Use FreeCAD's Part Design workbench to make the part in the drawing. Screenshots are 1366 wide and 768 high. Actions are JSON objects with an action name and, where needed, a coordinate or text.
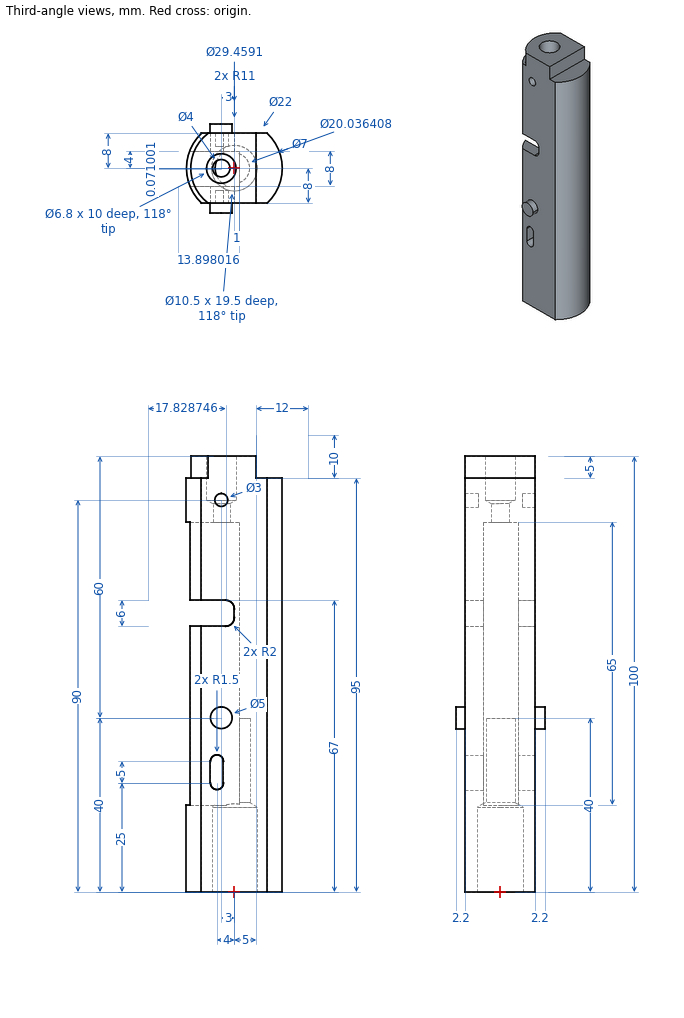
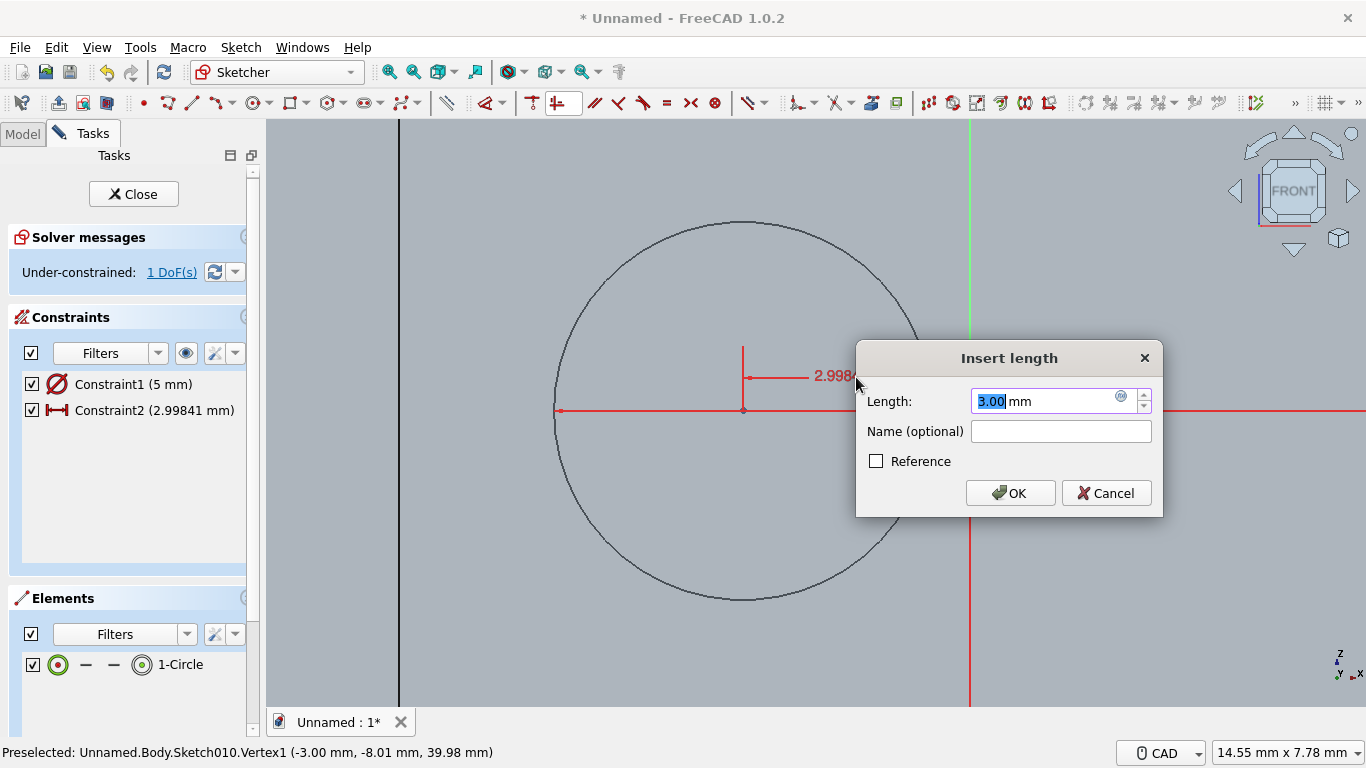
{"action": "type", "text": "3"}
{"action": "key", "text": "Return"}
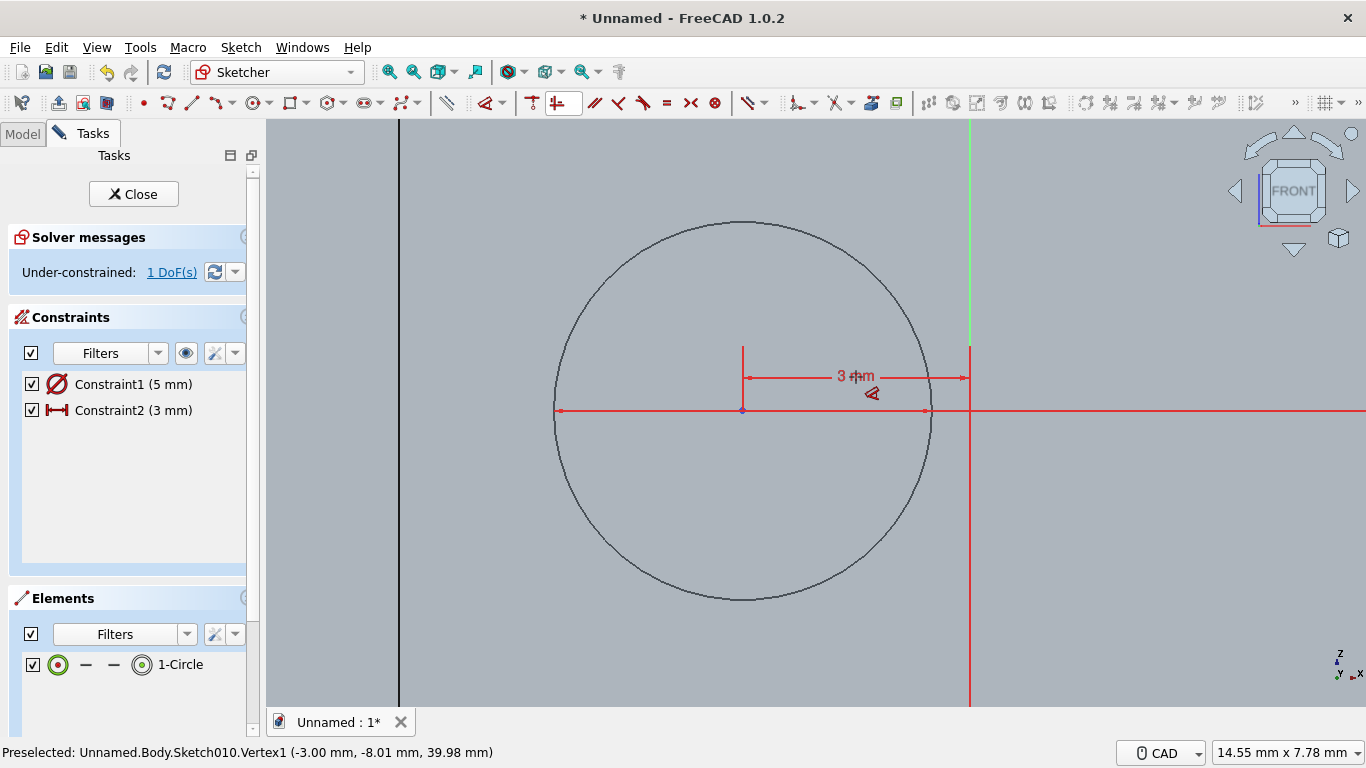
{"action": "left_click", "coordinate": [743, 411]}
{"action": "left_click", "coordinate": [1004, 545]}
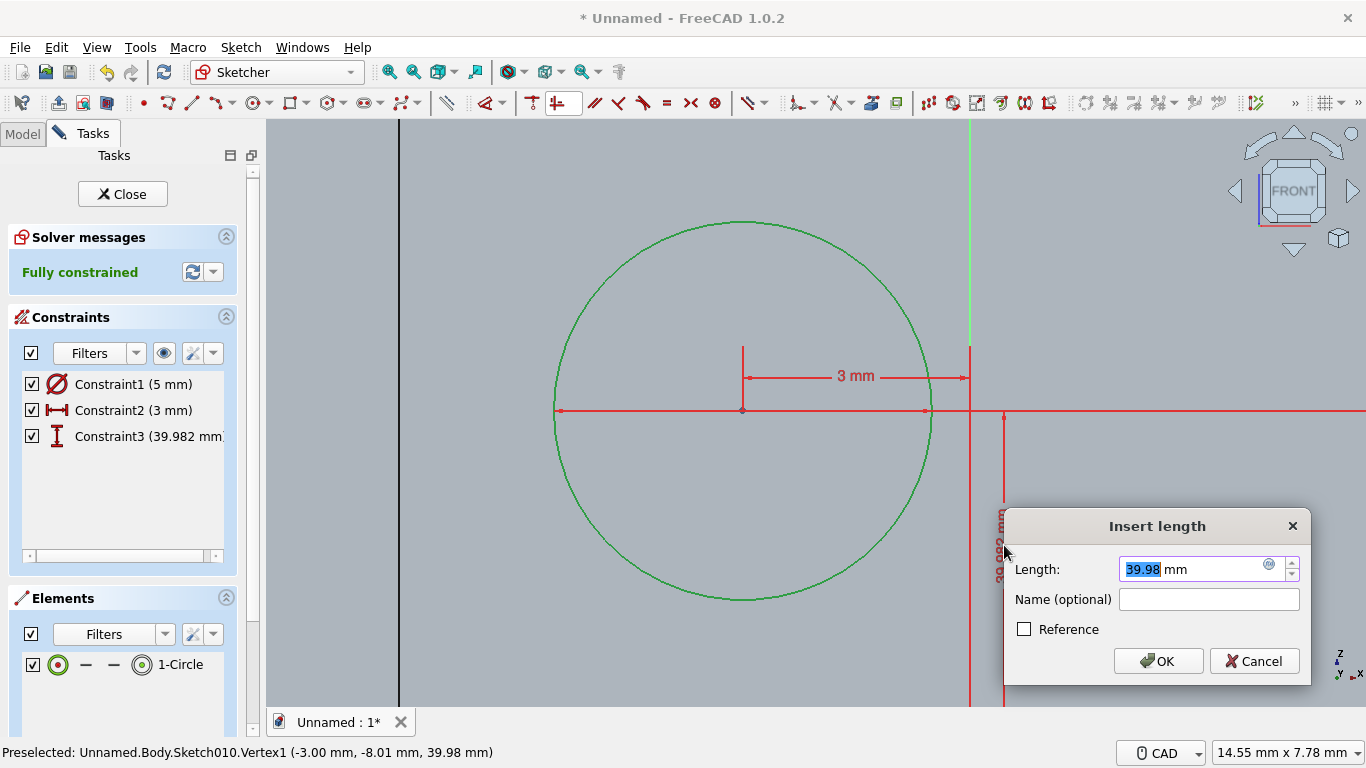
{"action": "type", "text": "40"}
{"action": "key", "text": "Return"}
{"action": "key", "text": "Escape"}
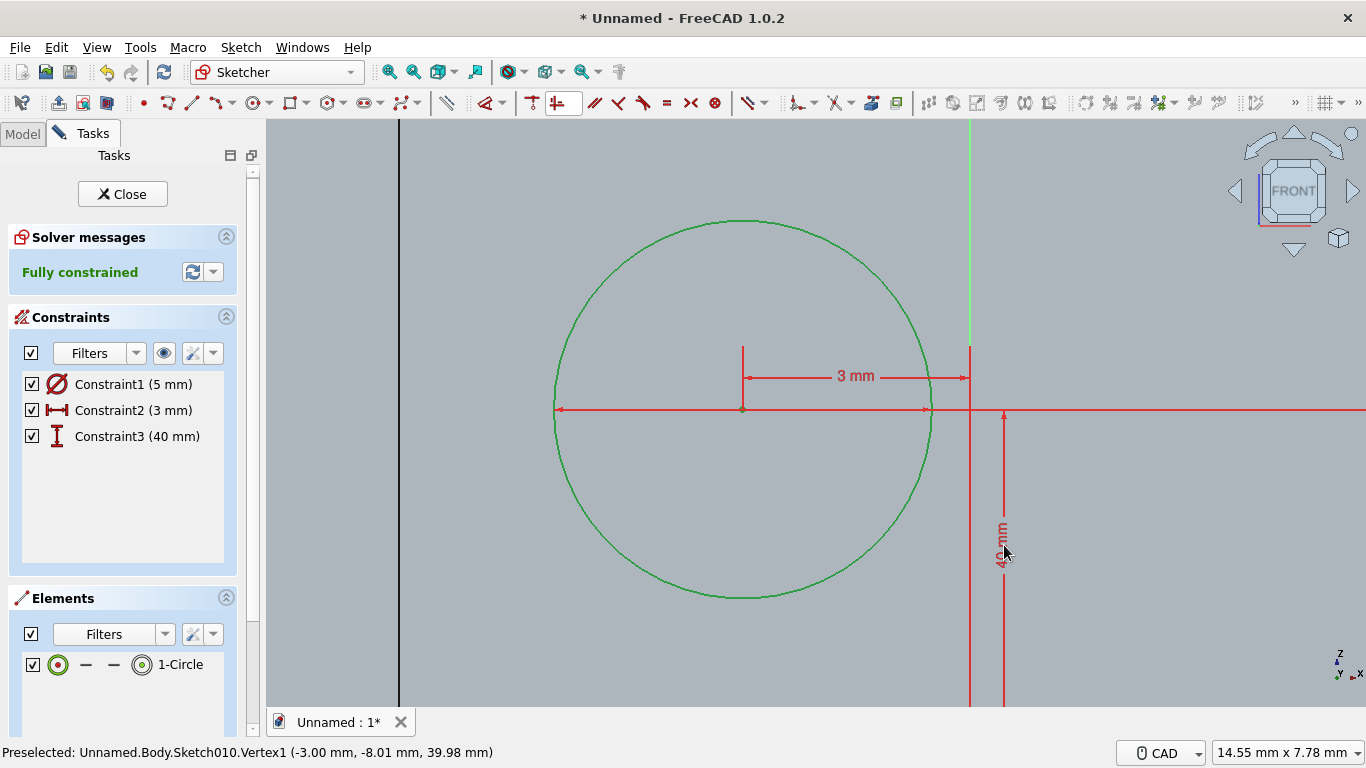
{"action": "left_click", "coordinate": [123, 194]}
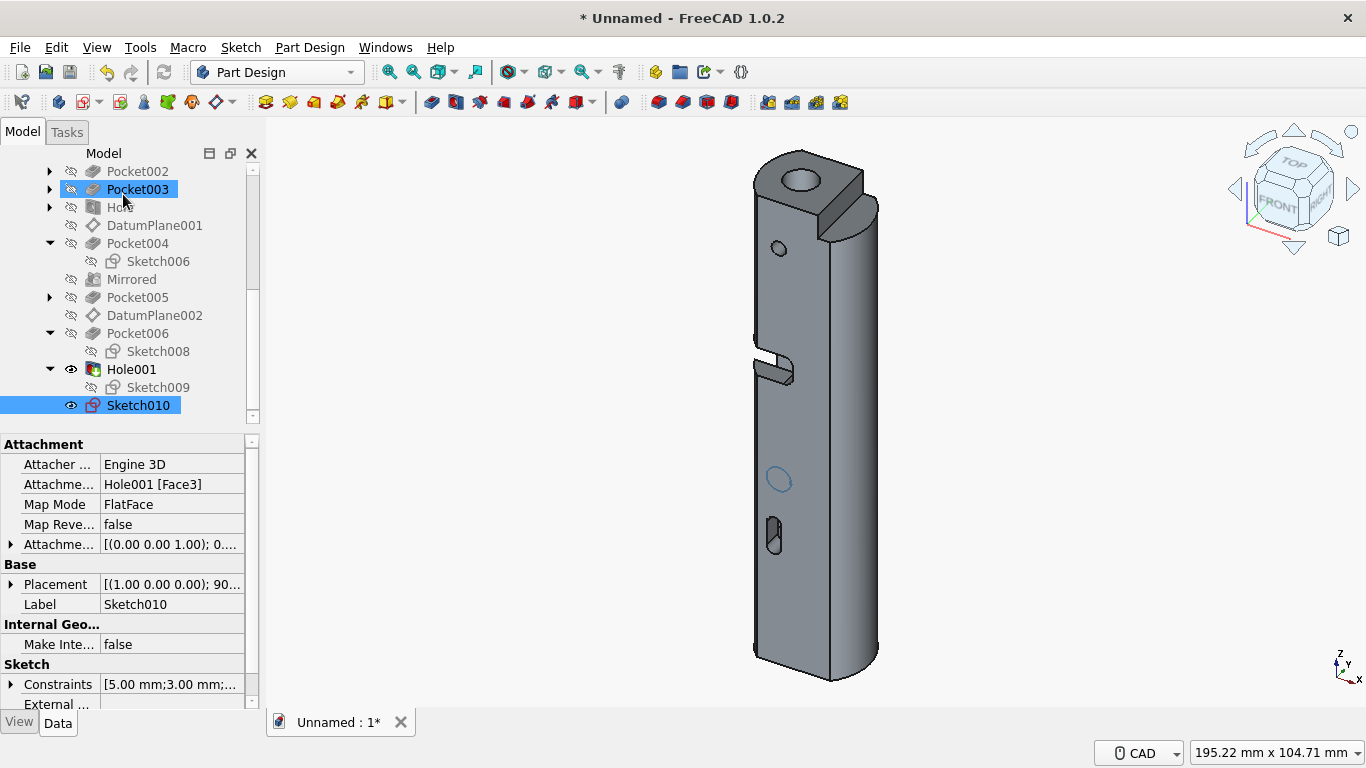
{"action": "left_click", "coordinate": [266, 102]}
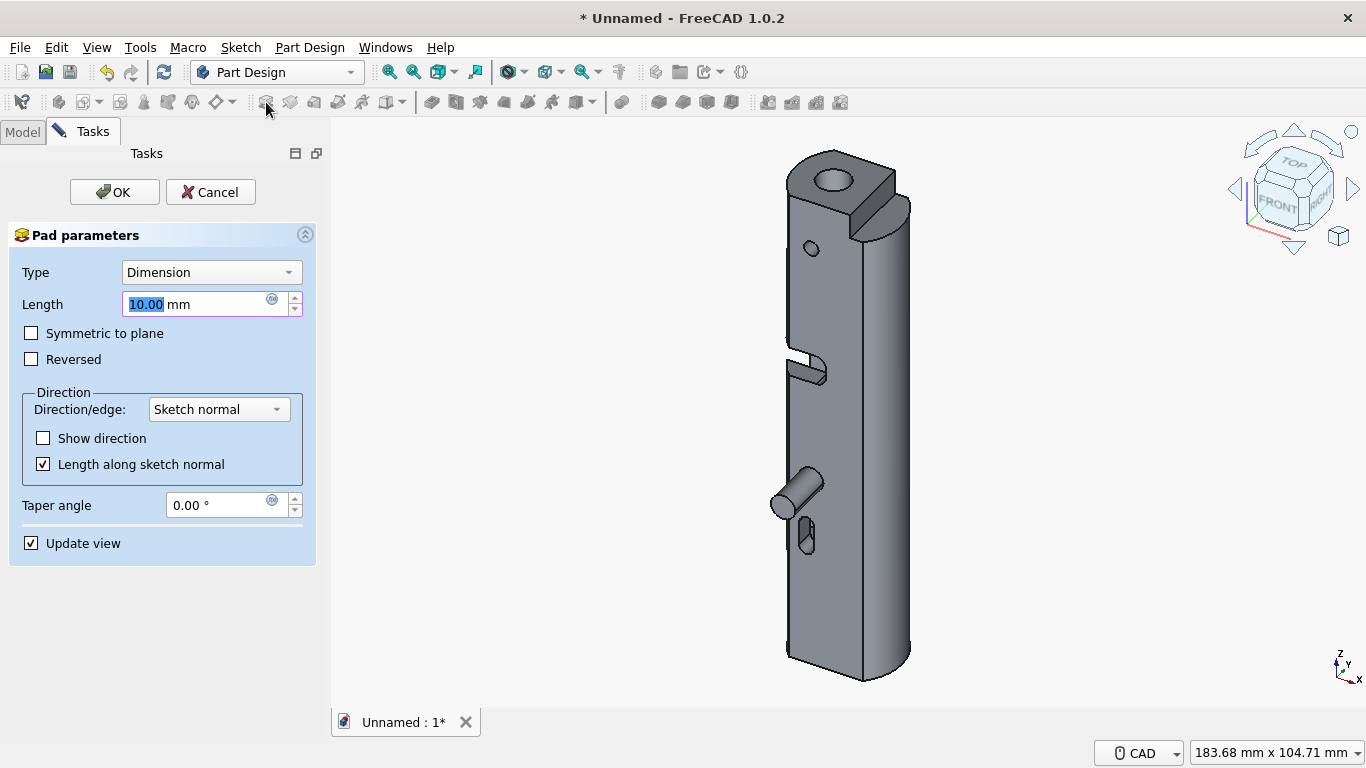
{"action": "type", "text": "2.2"}
{"action": "key", "text": "Tab"}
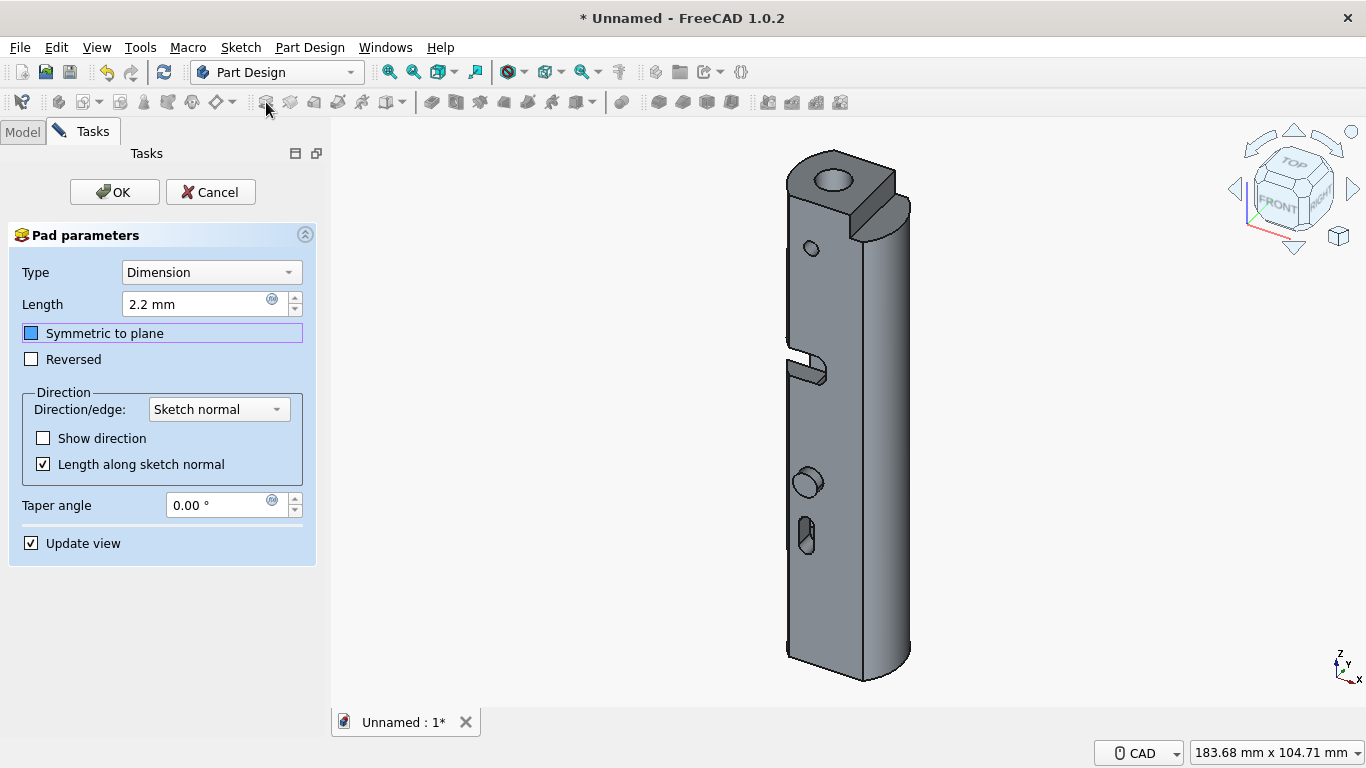
{"action": "left_click", "coordinate": [115, 192]}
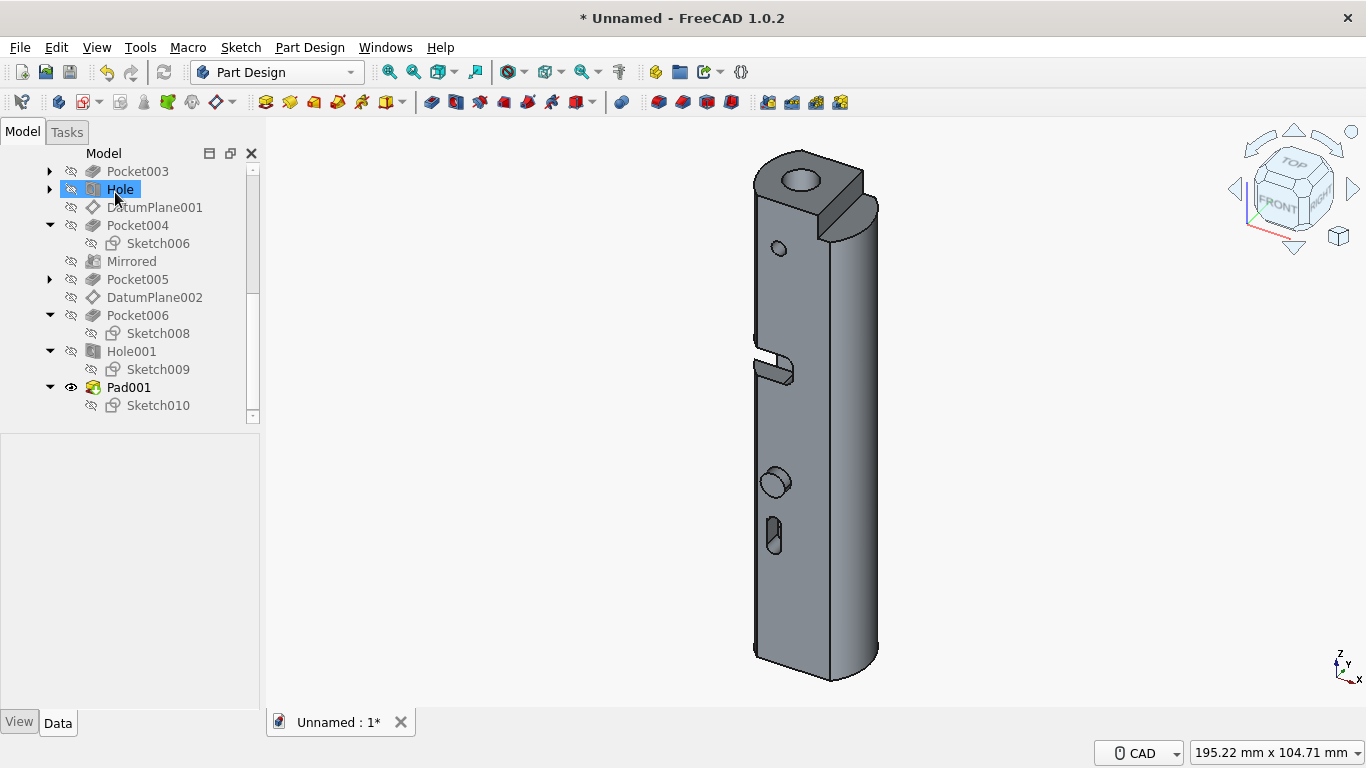
{"action": "scroll", "coordinate": [140, 293], "scroll_direction": "down", "scroll_amount": 3}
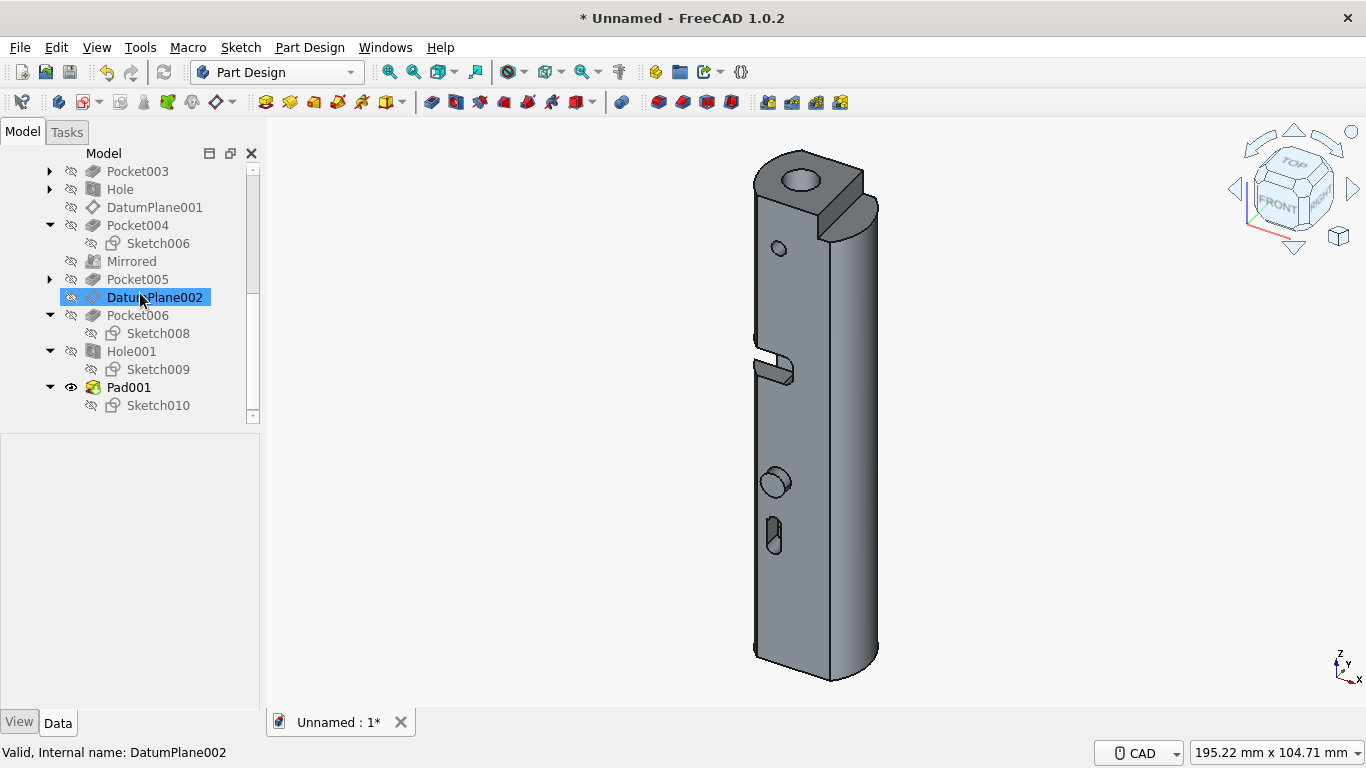
{"action": "scroll", "coordinate": [140, 293], "scroll_direction": "up", "scroll_amount": 15}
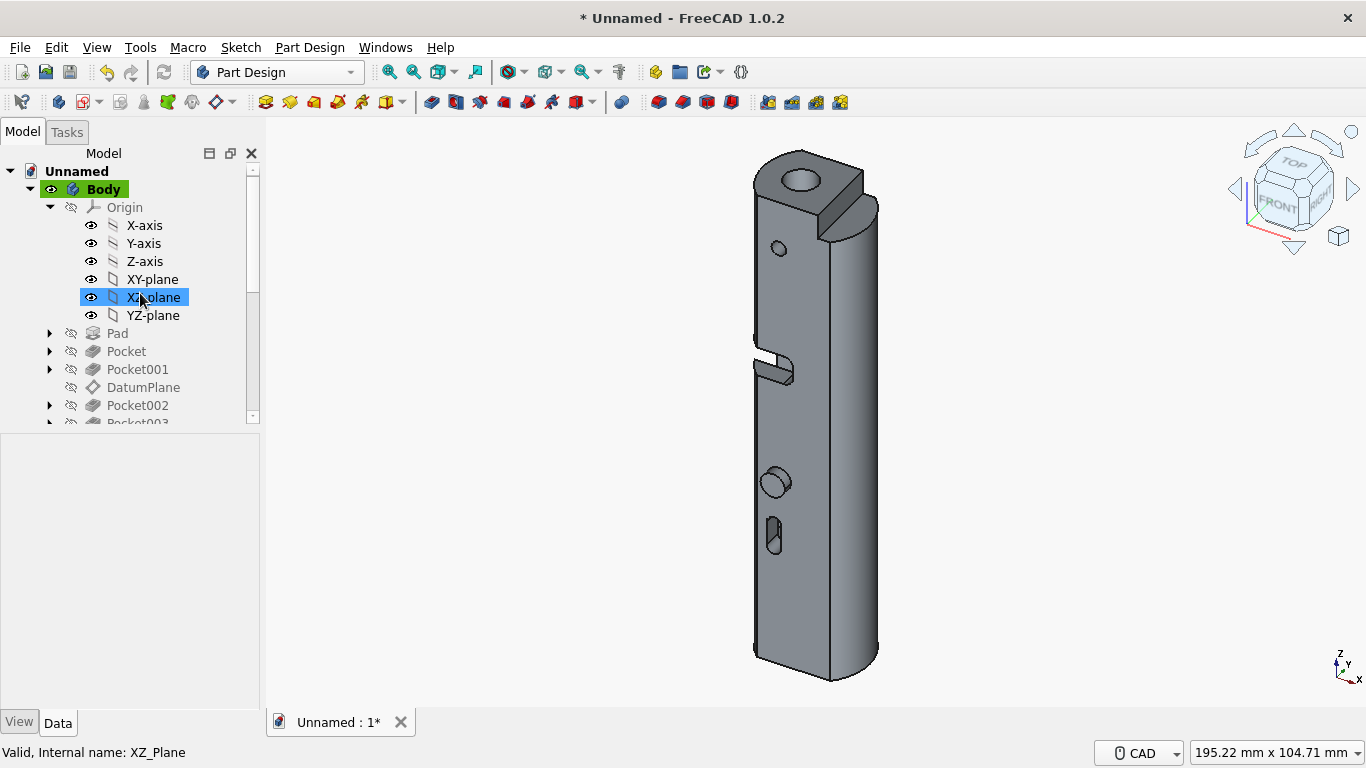
{"action": "left_click", "coordinate": [136, 297]}